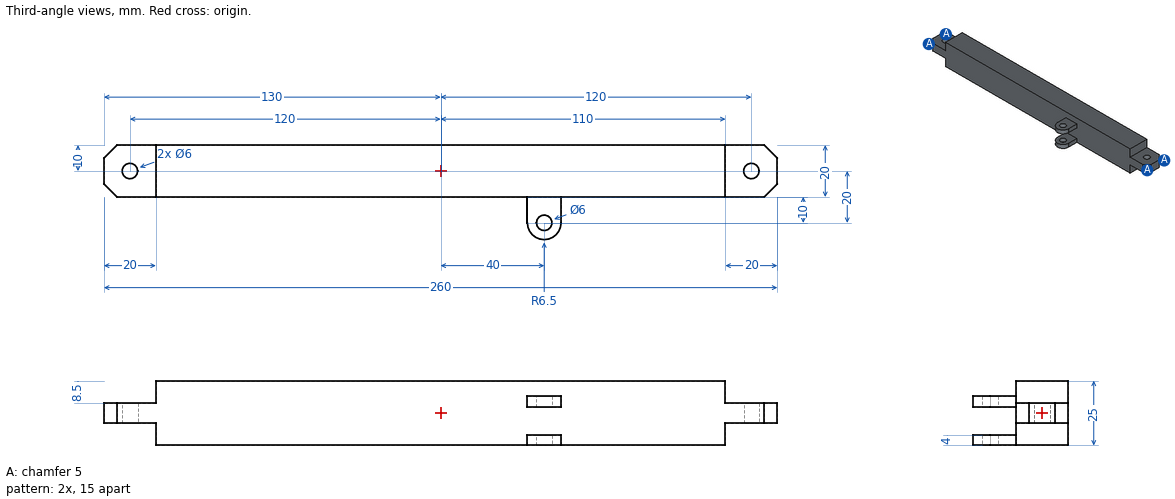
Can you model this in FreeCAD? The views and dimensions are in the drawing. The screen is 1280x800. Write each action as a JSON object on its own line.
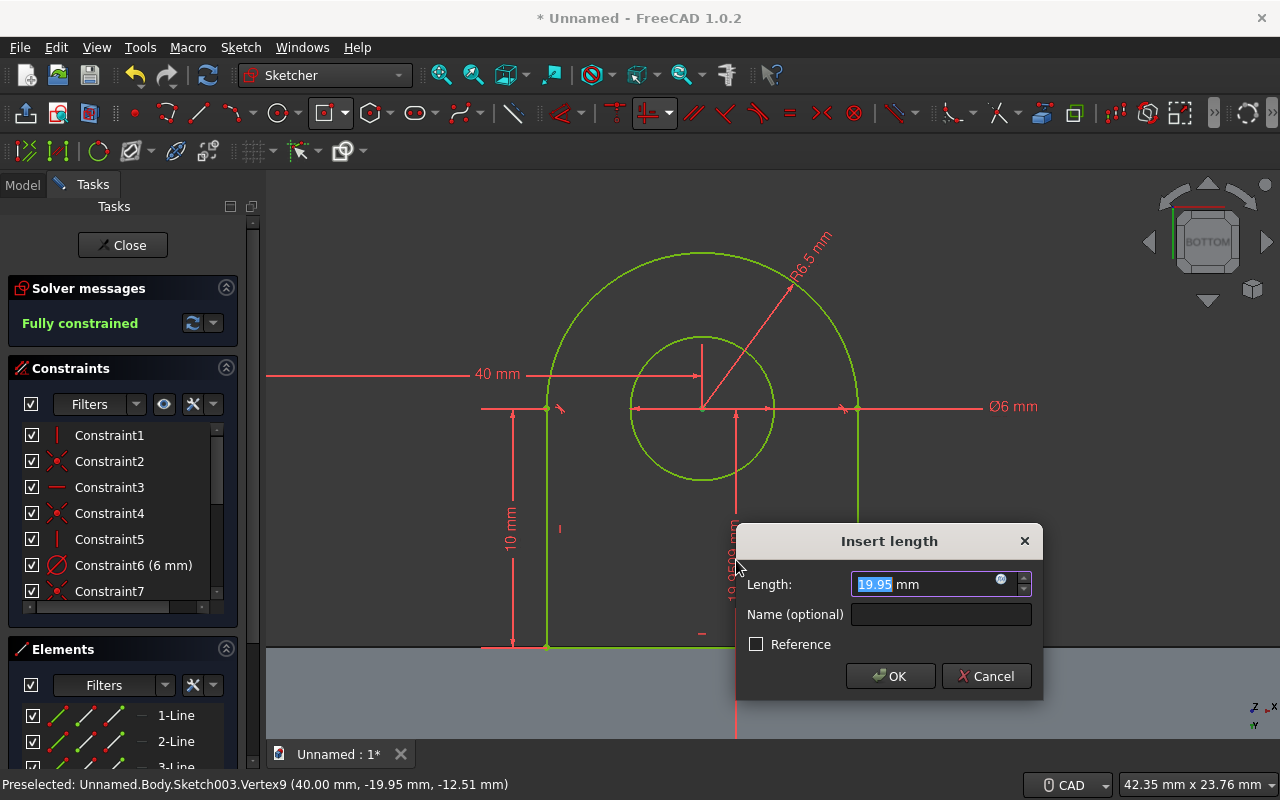
{"action": "type", "text": "20"}
{"action": "key", "text": "Return"}
{"action": "key", "text": "Escape"}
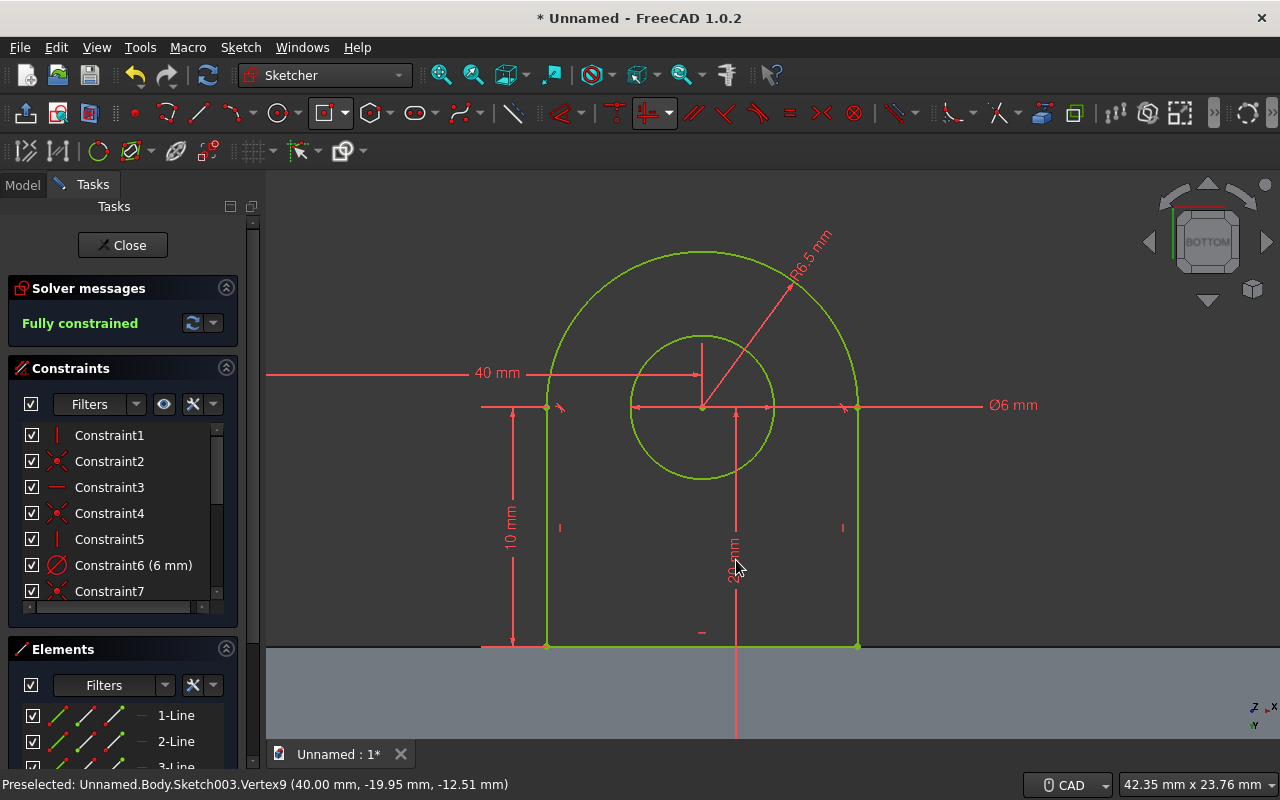
{"action": "left_click", "coordinate": [123, 245]}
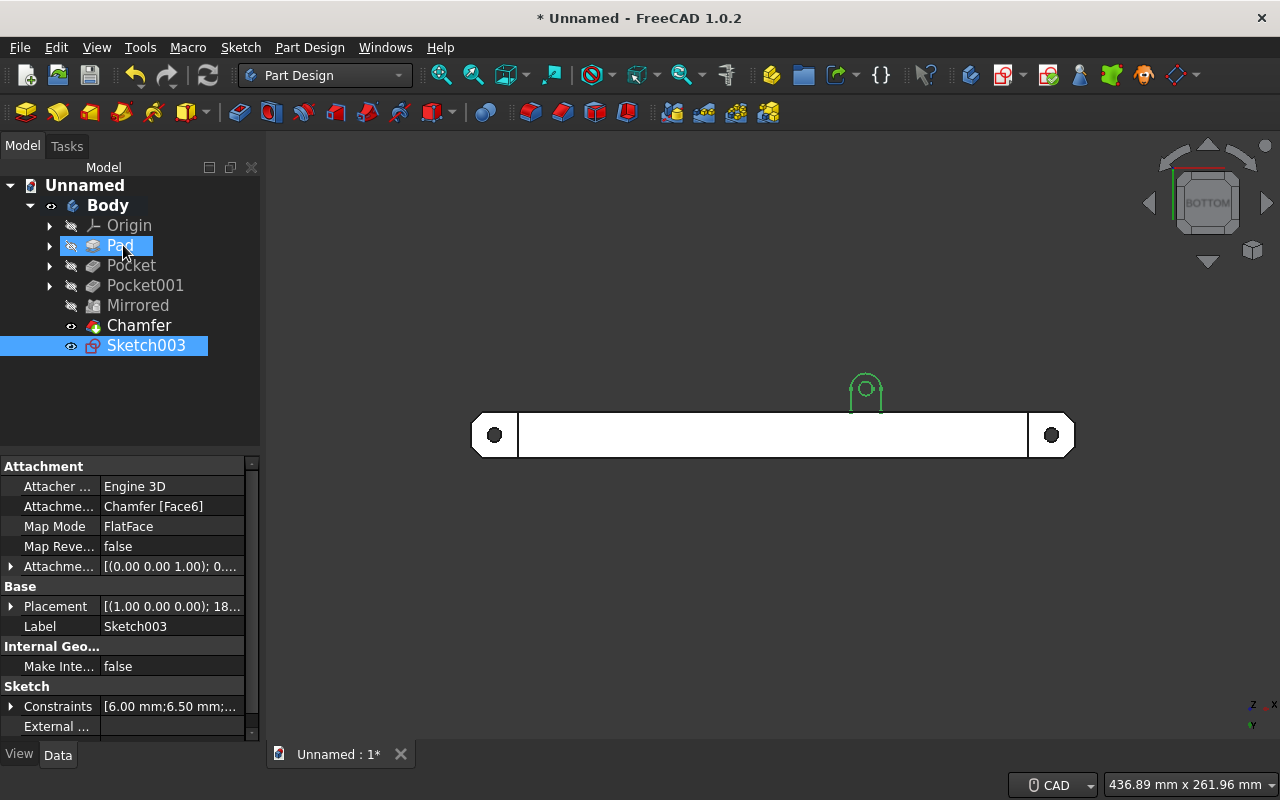
{"action": "left_click", "coordinate": [26, 112]}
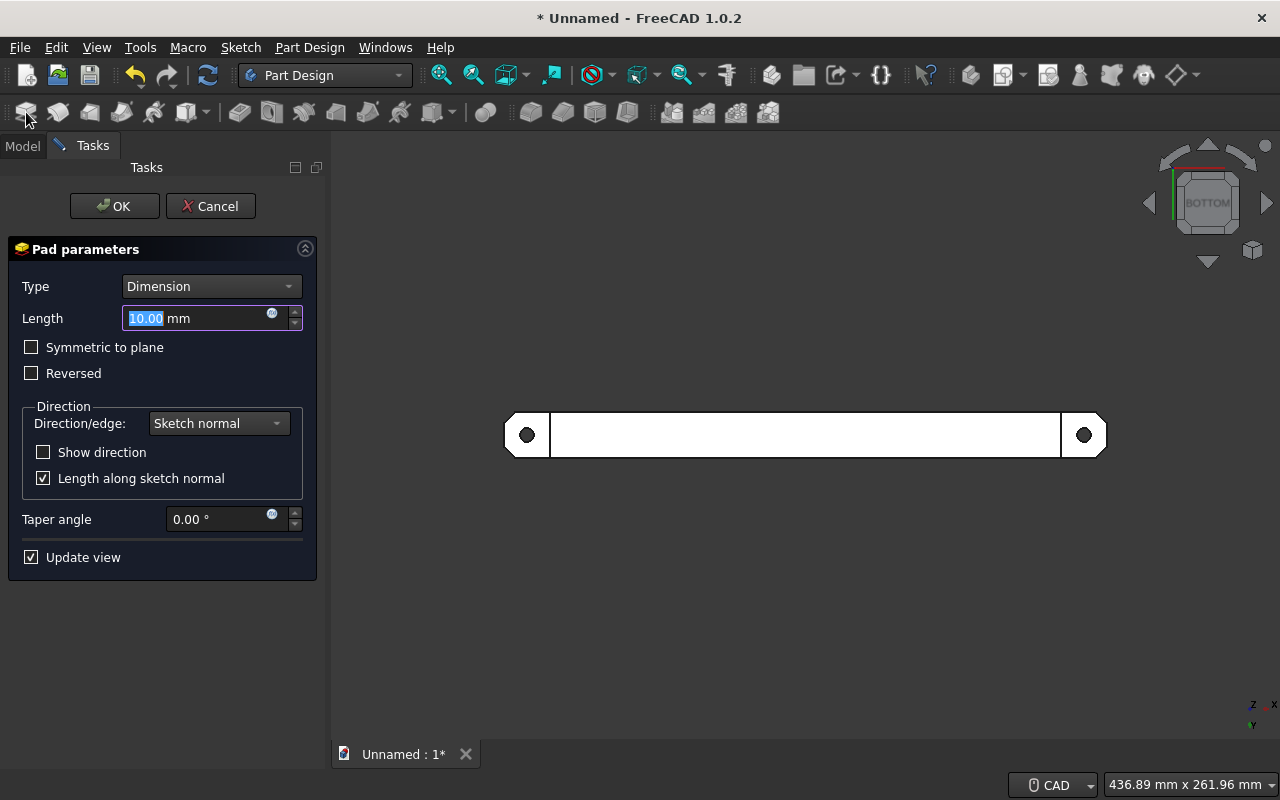
{"action": "type", "text": "4"}
{"action": "key", "text": "Tab"}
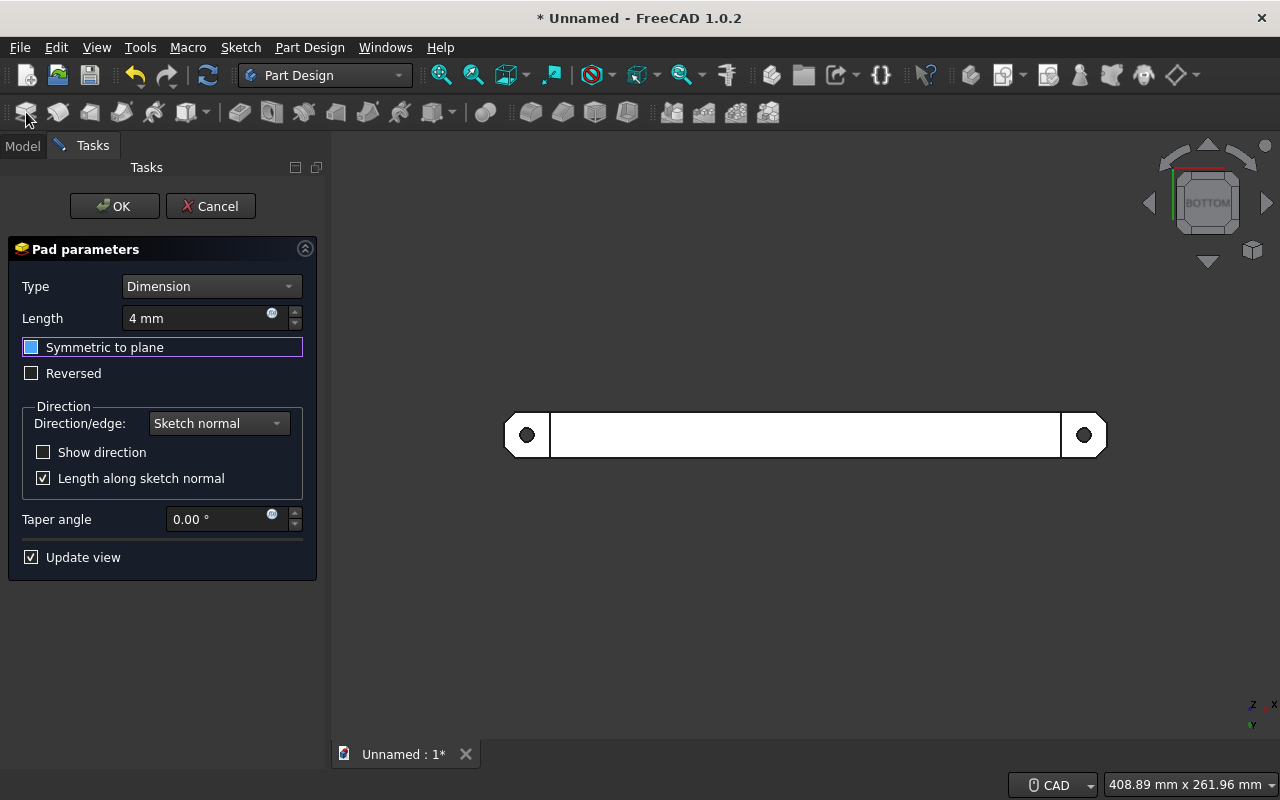
{"action": "left_click", "coordinate": [30, 373]}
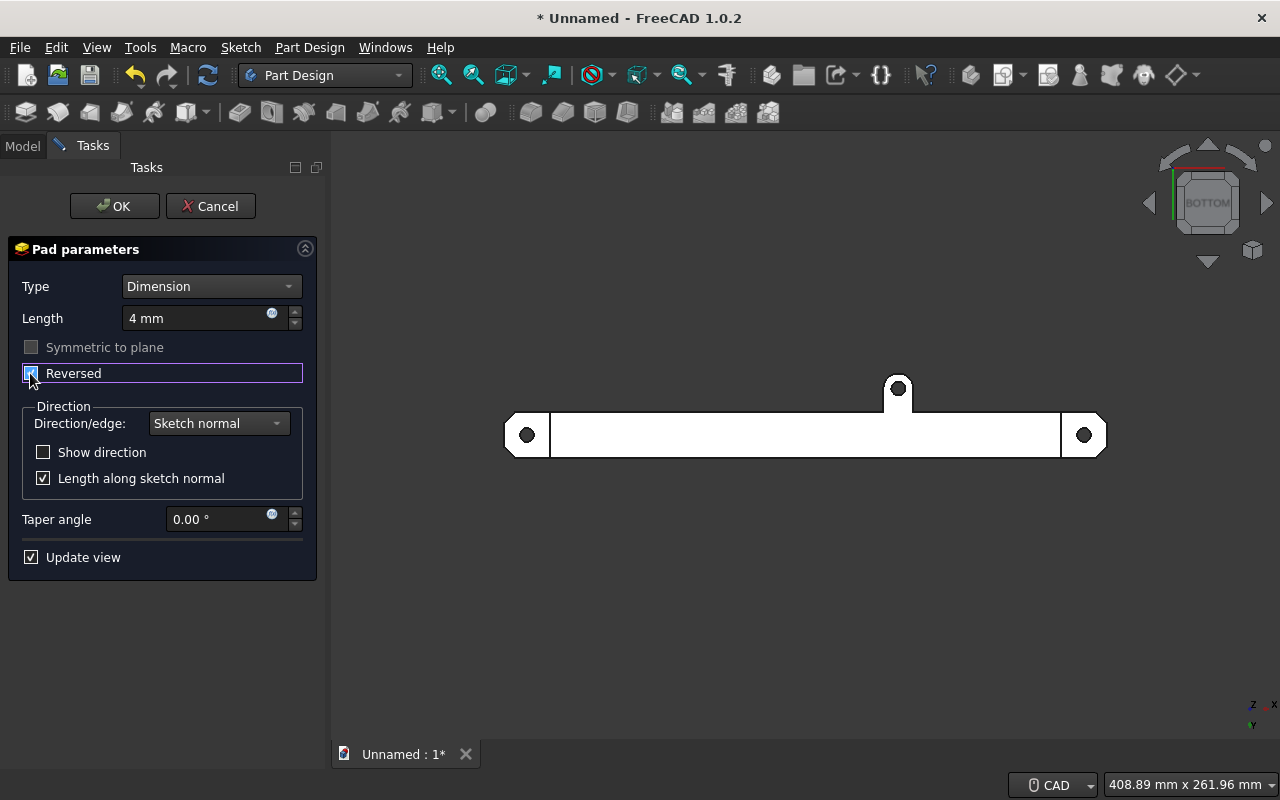
{"action": "left_click", "coordinate": [115, 206]}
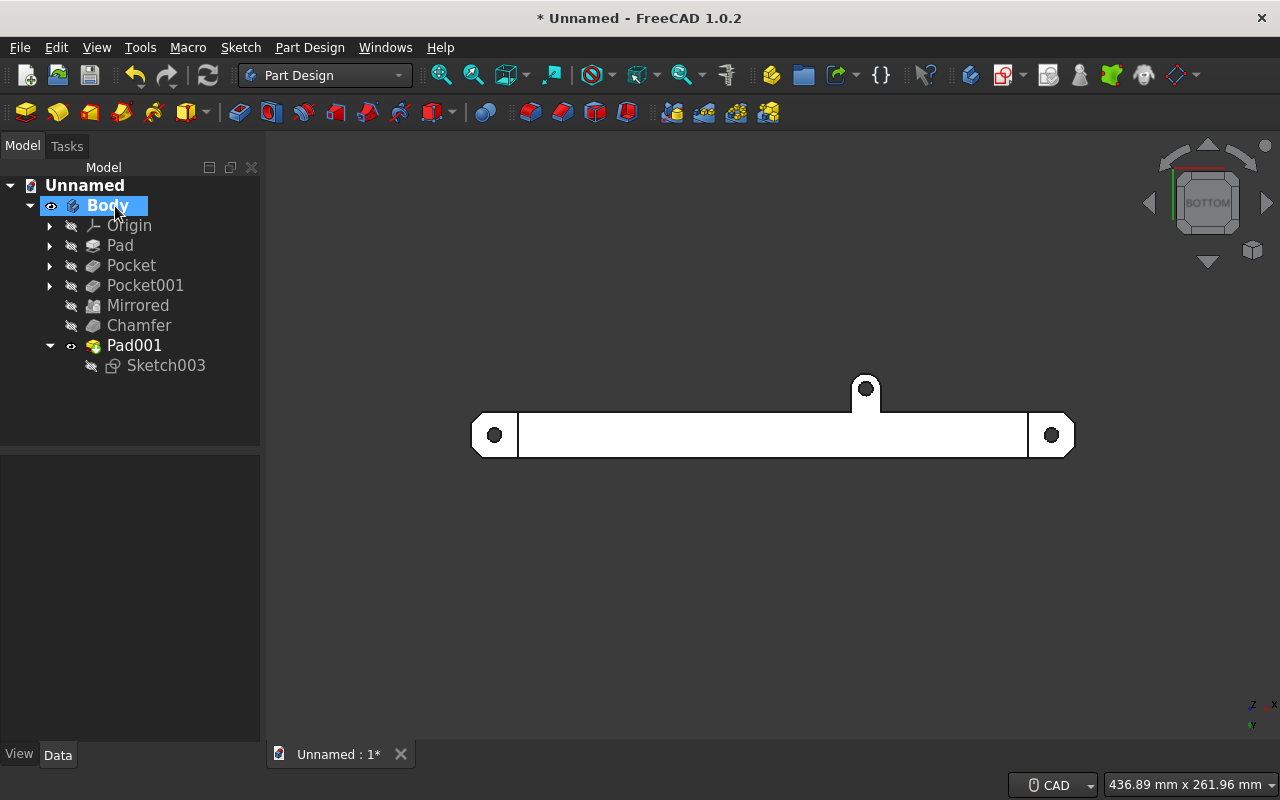
{"action": "left_click", "coordinate": [116, 346]}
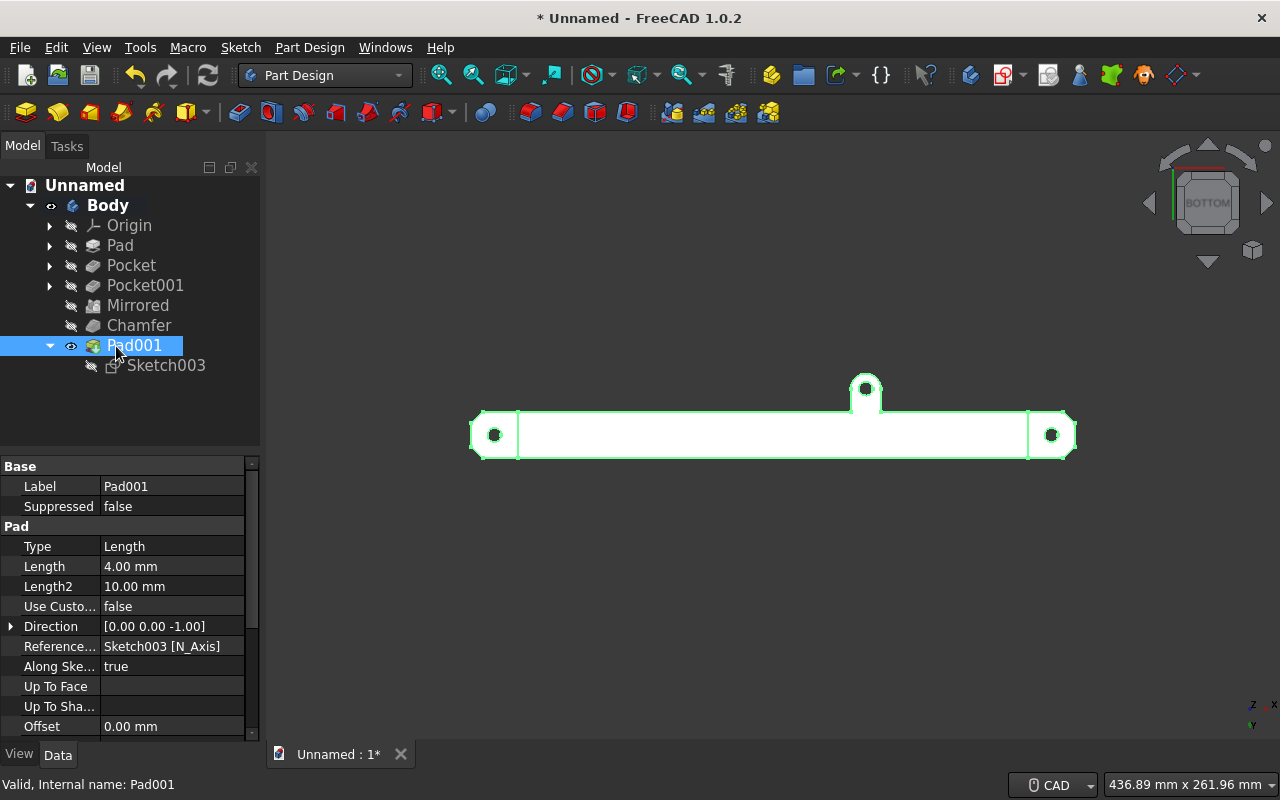
{"action": "left_click", "coordinate": [704, 112]}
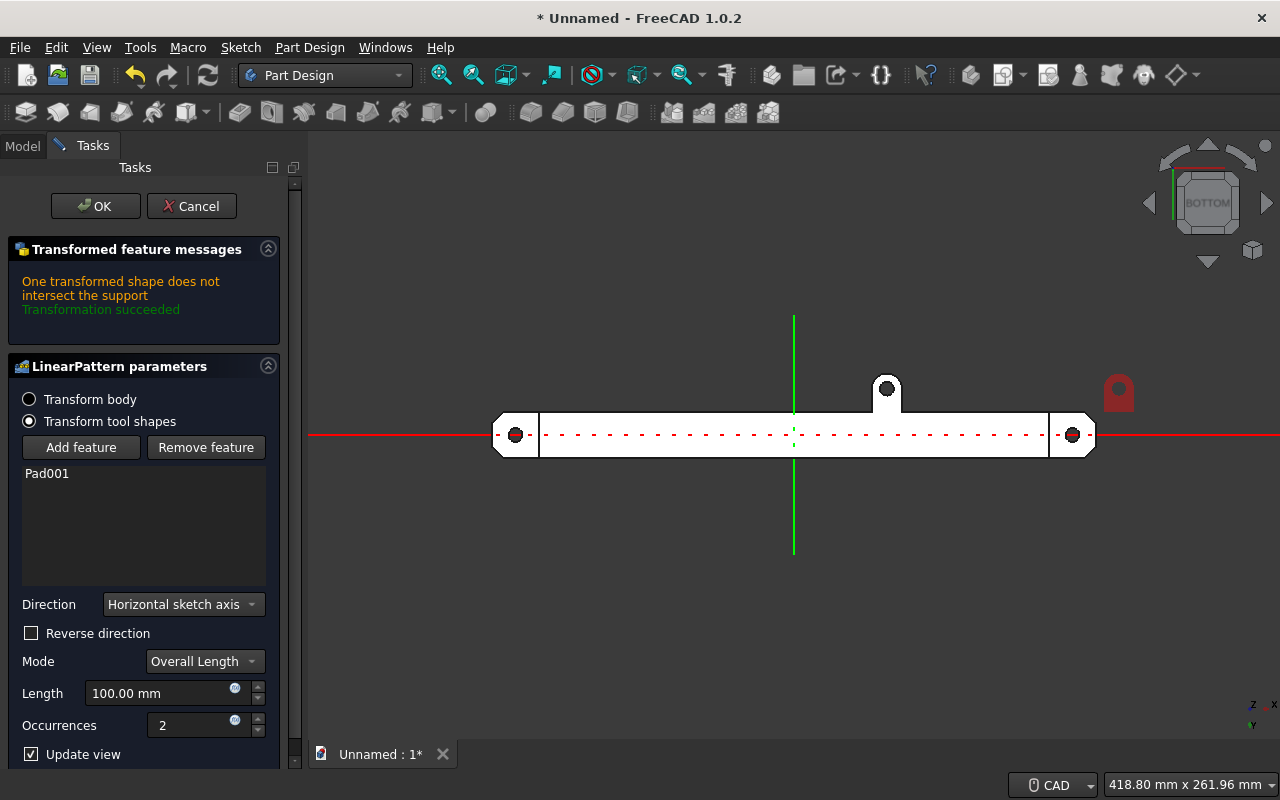
{"action": "left_click", "coordinate": [184, 604]}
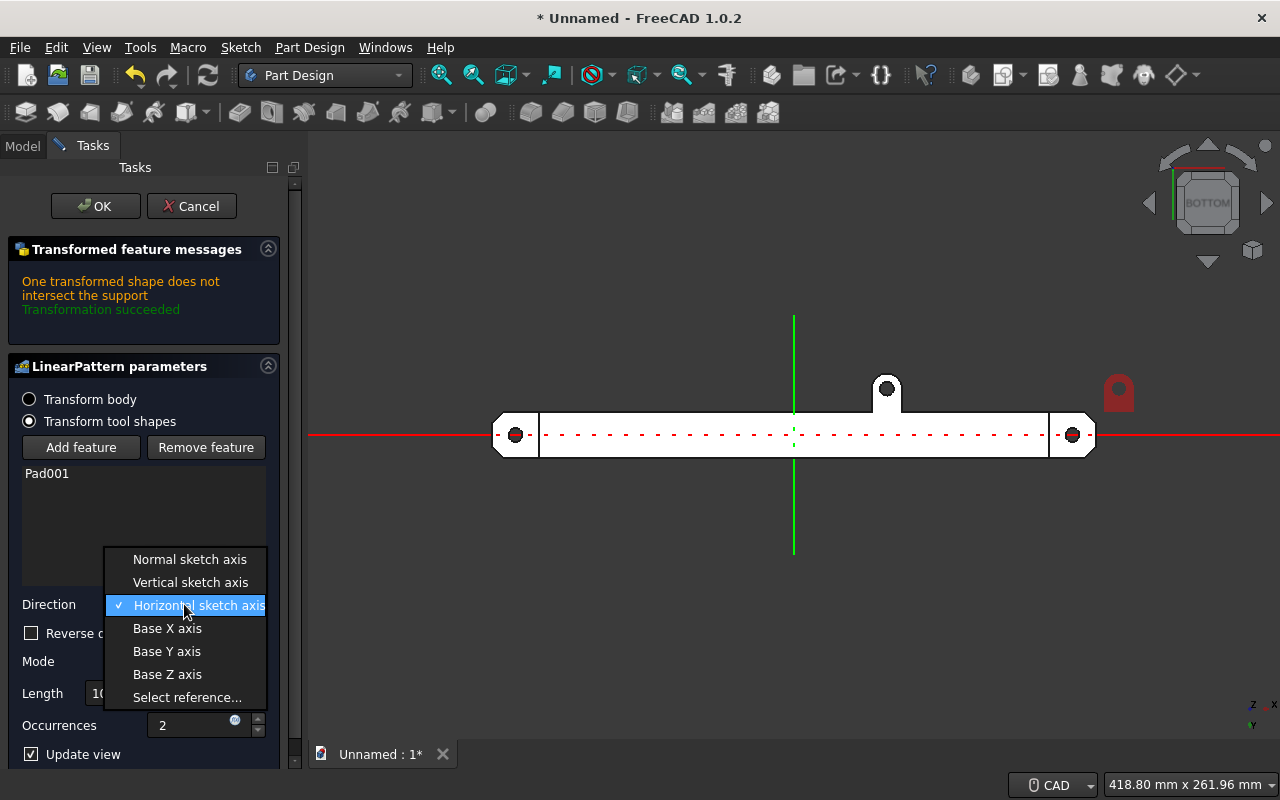
{"action": "left_click", "coordinate": [184, 674]}